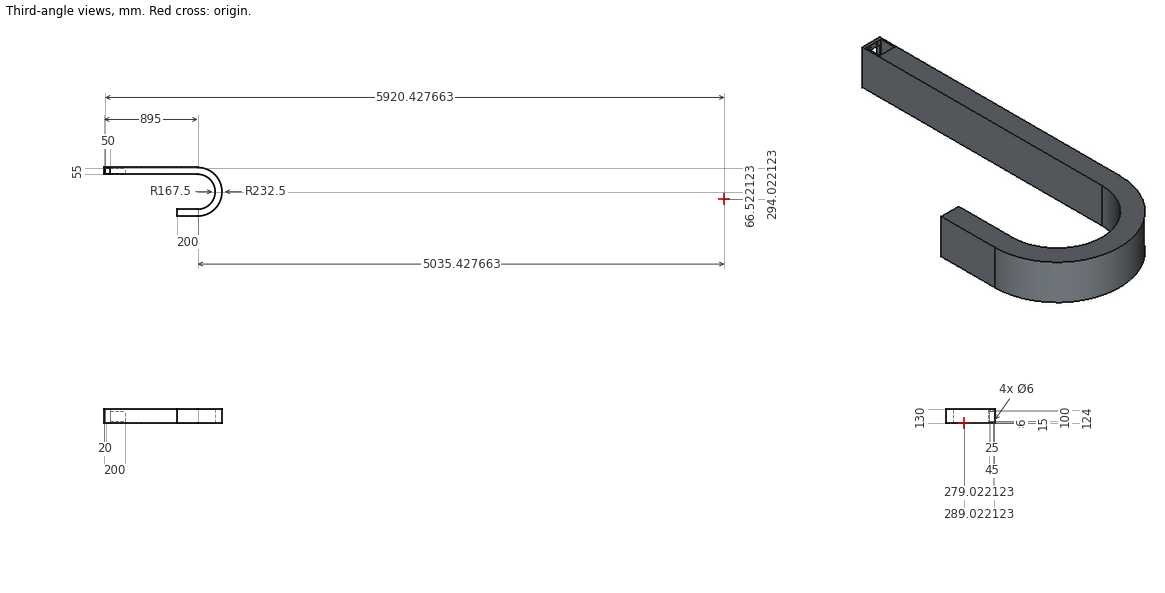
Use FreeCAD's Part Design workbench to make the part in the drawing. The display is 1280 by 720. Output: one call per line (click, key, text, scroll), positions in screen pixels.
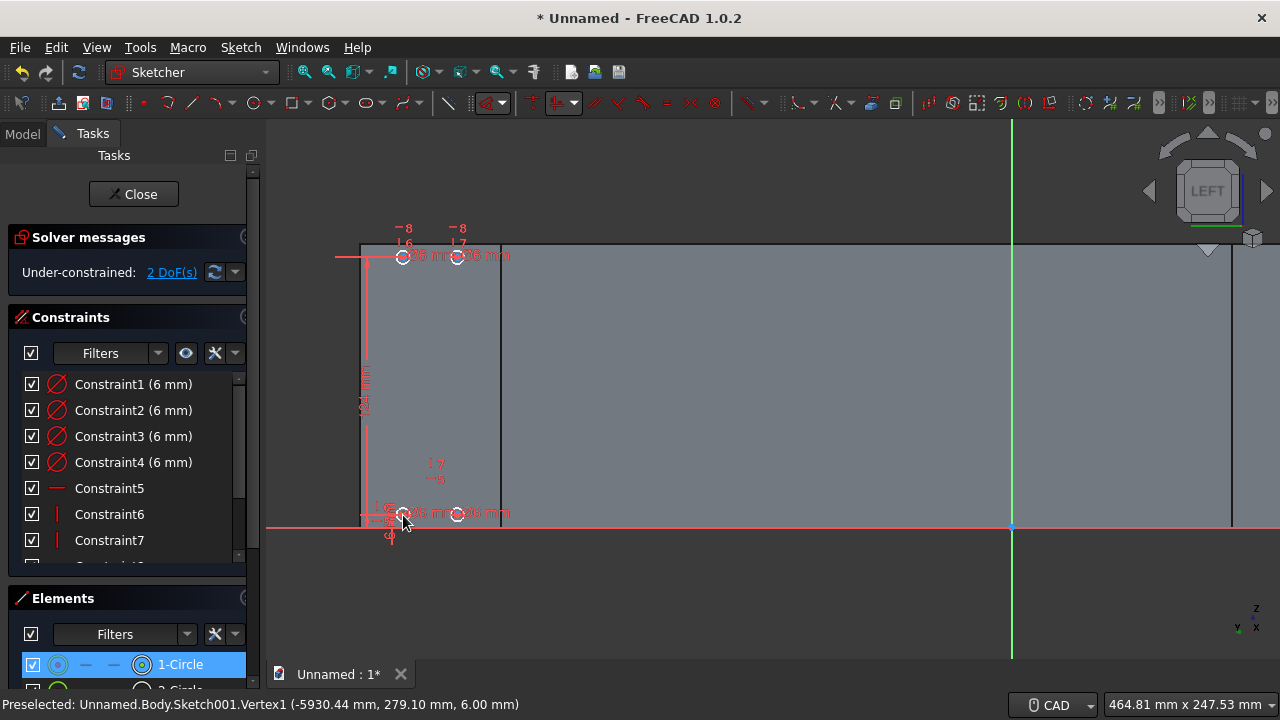
click(457, 515)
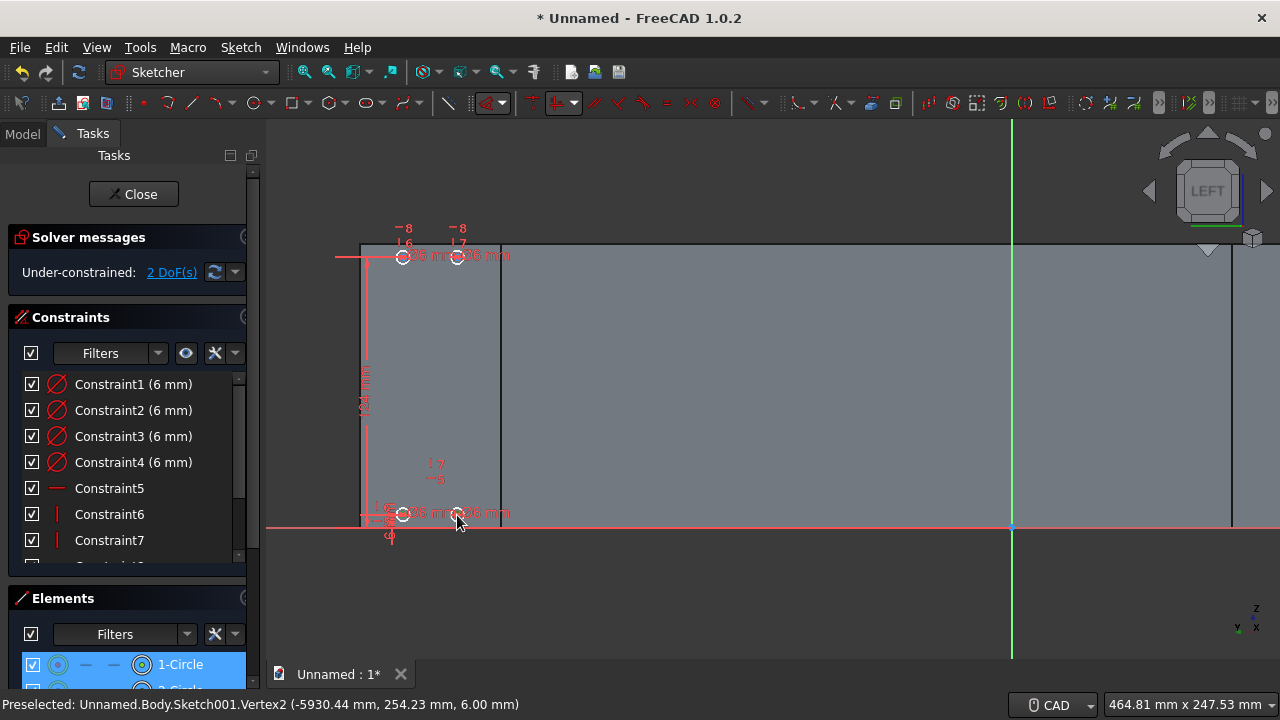
key(l)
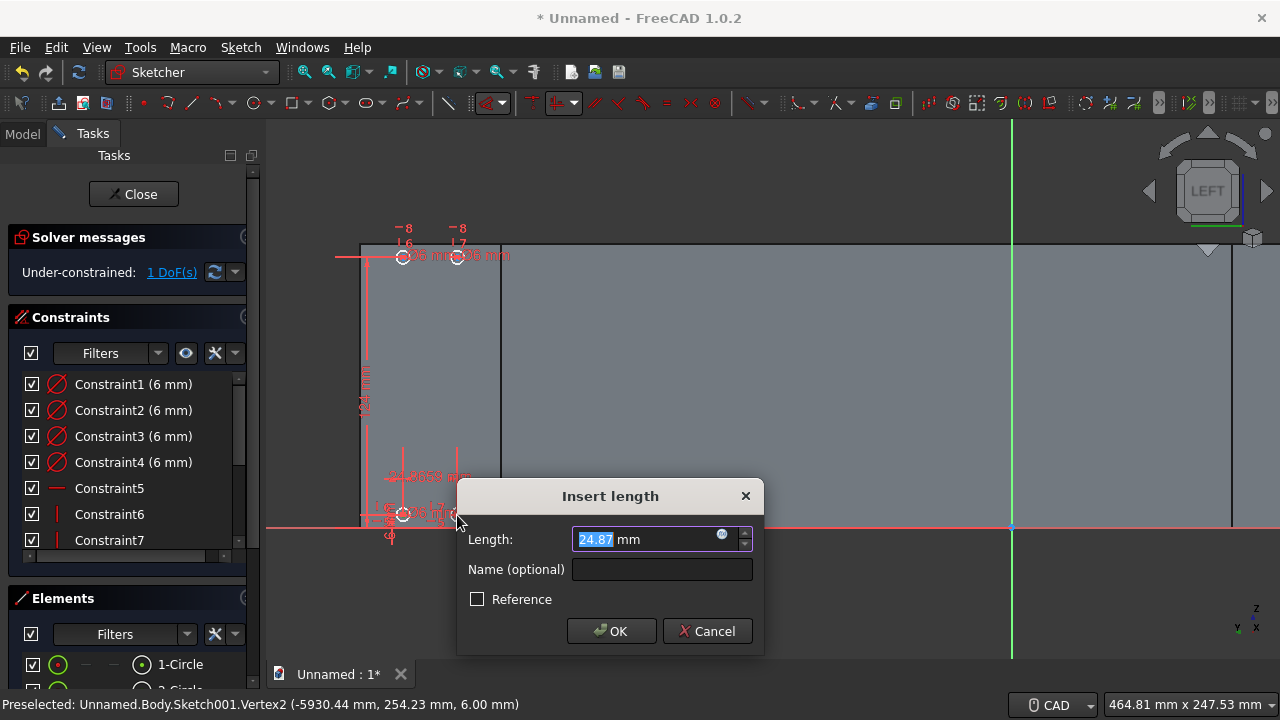
text(25)
key(Return)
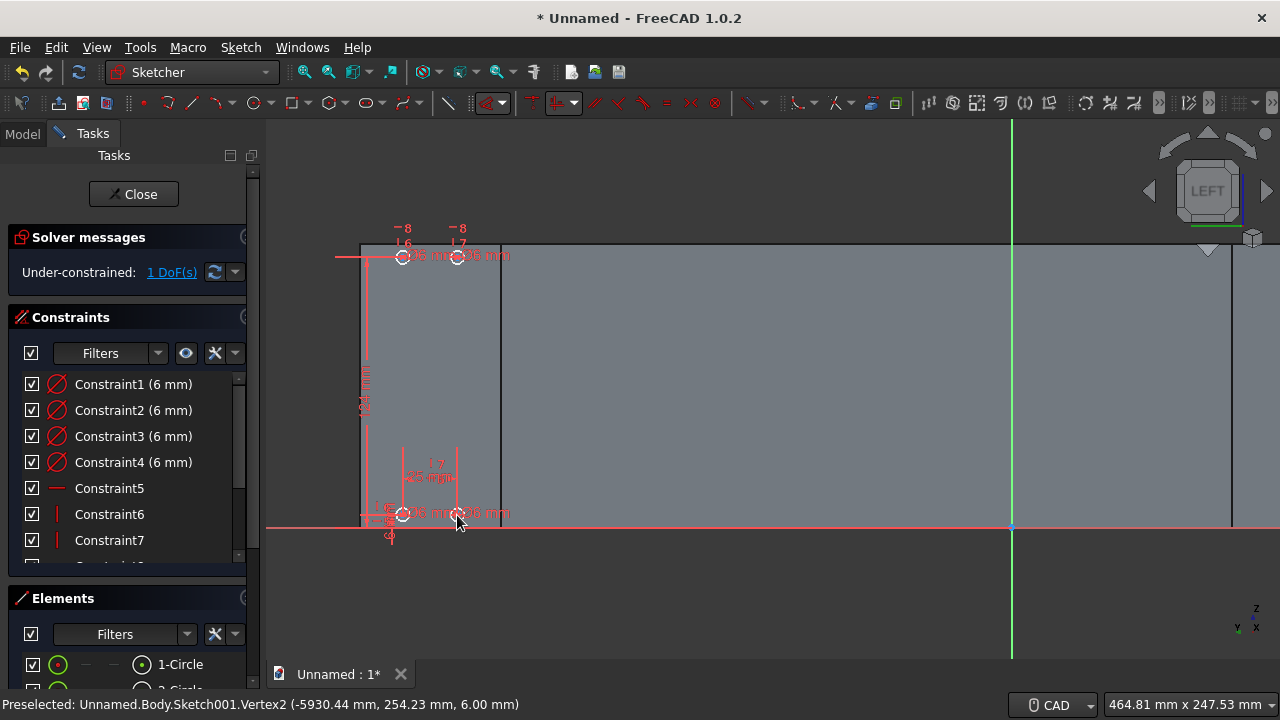
click(403, 515)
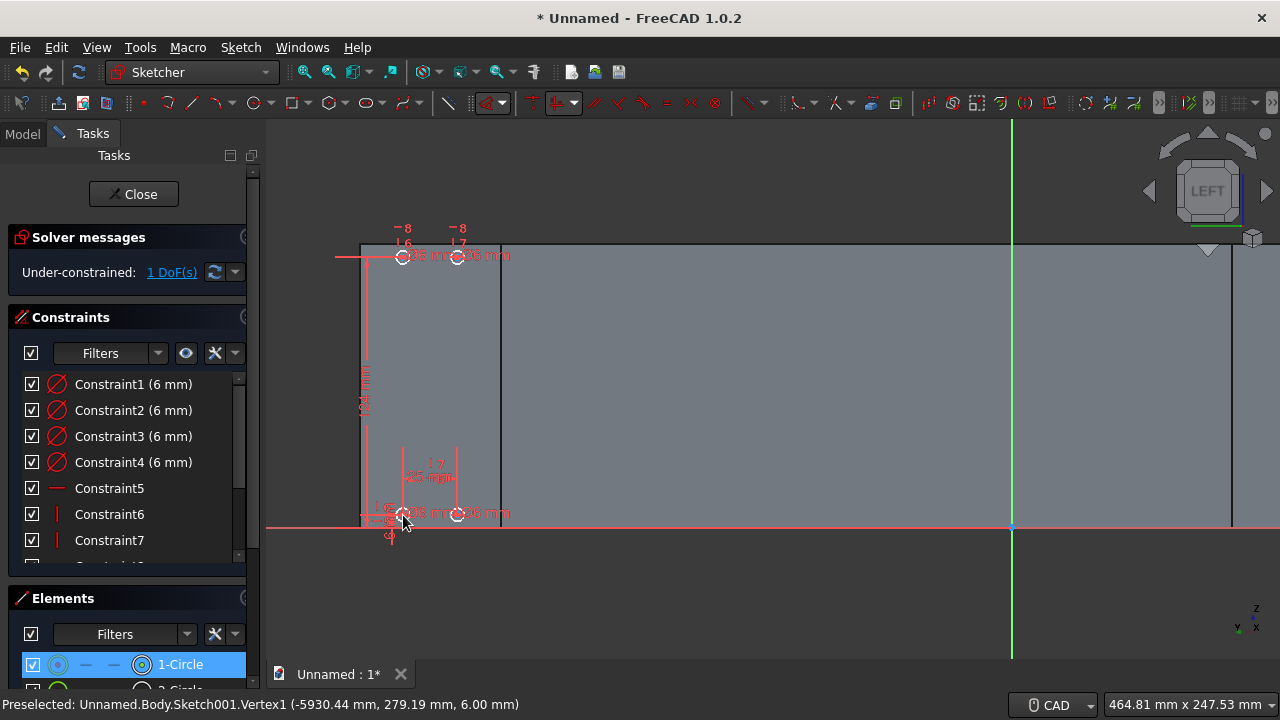
key(l)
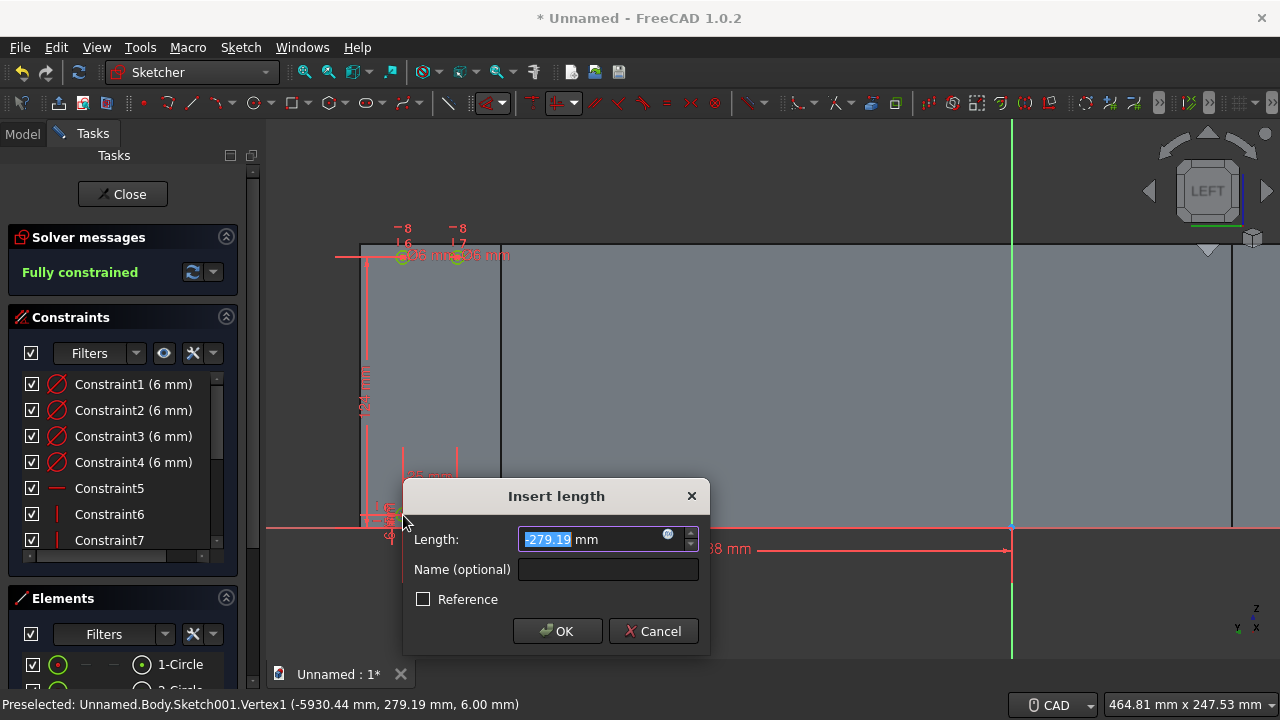
text(-279.022123)
key(Return)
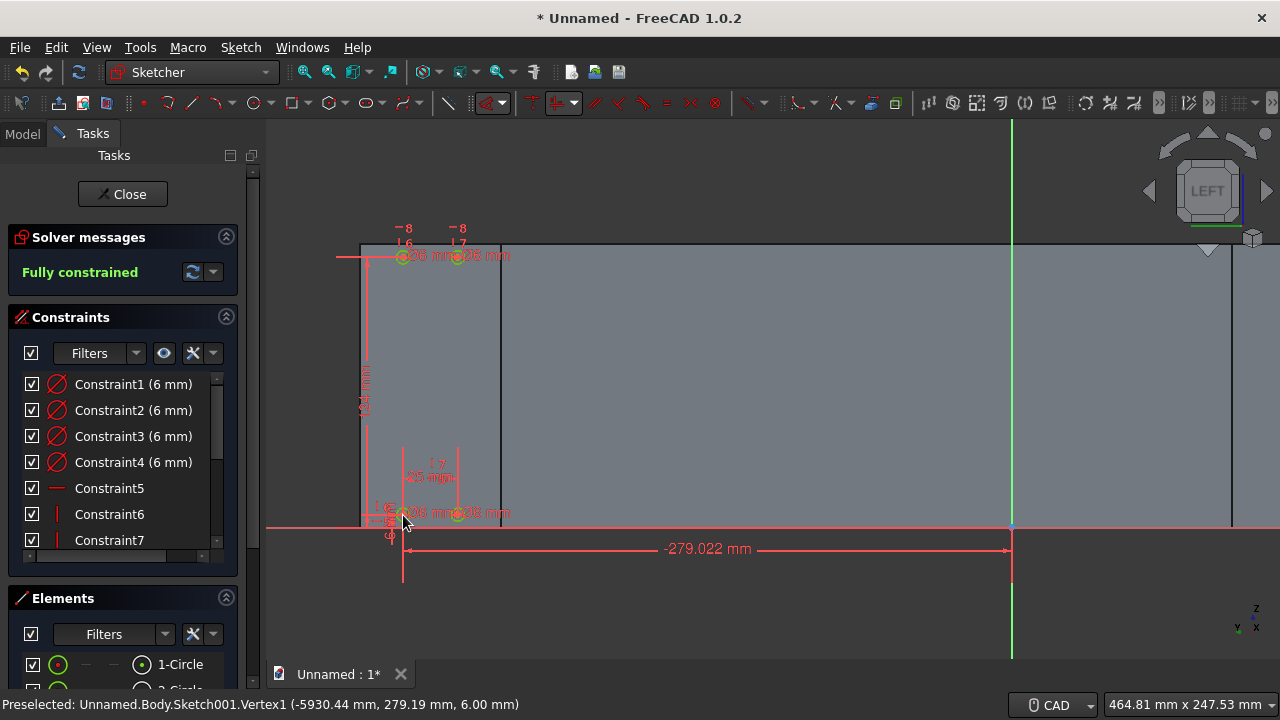
click(123, 194)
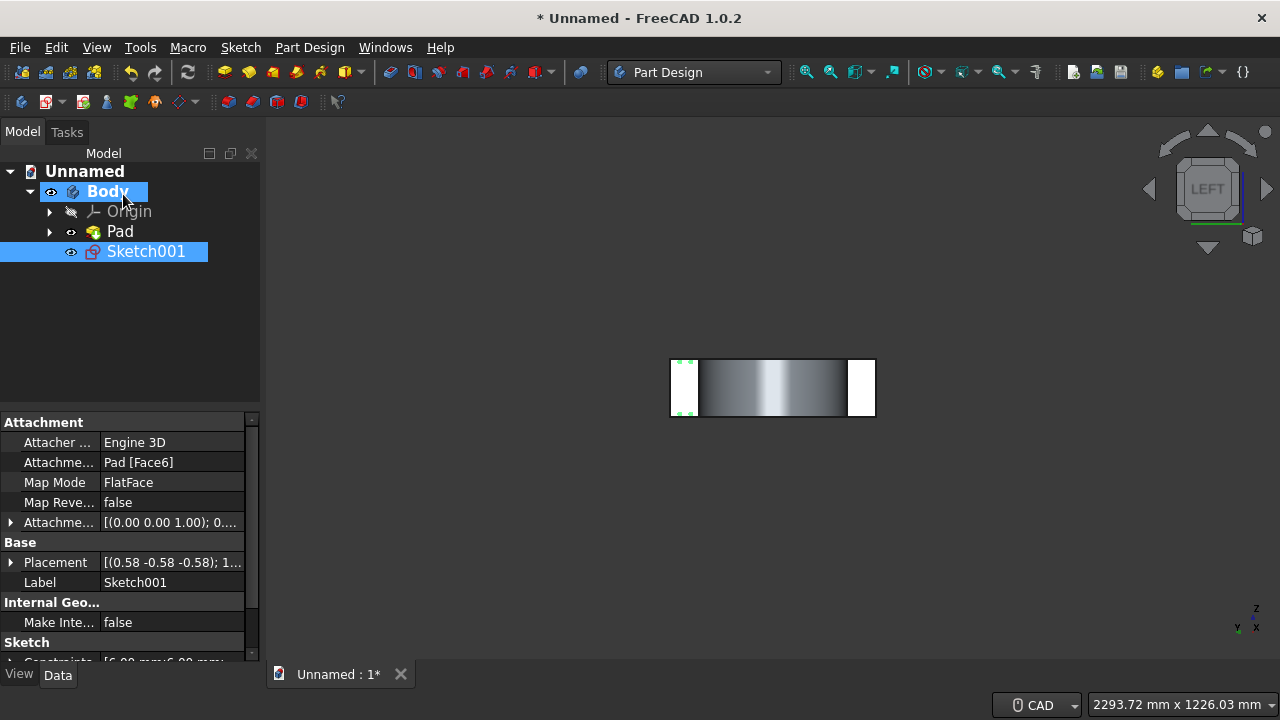
click(392, 72)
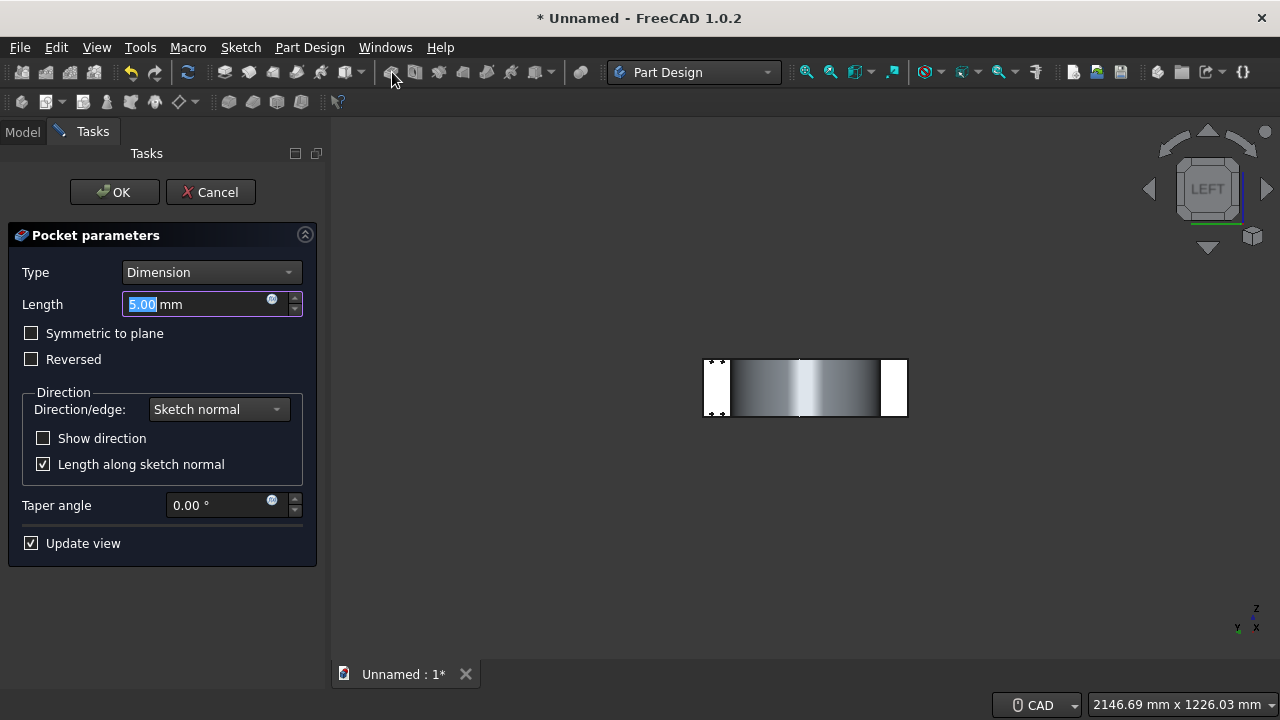
text(20)
key(Tab)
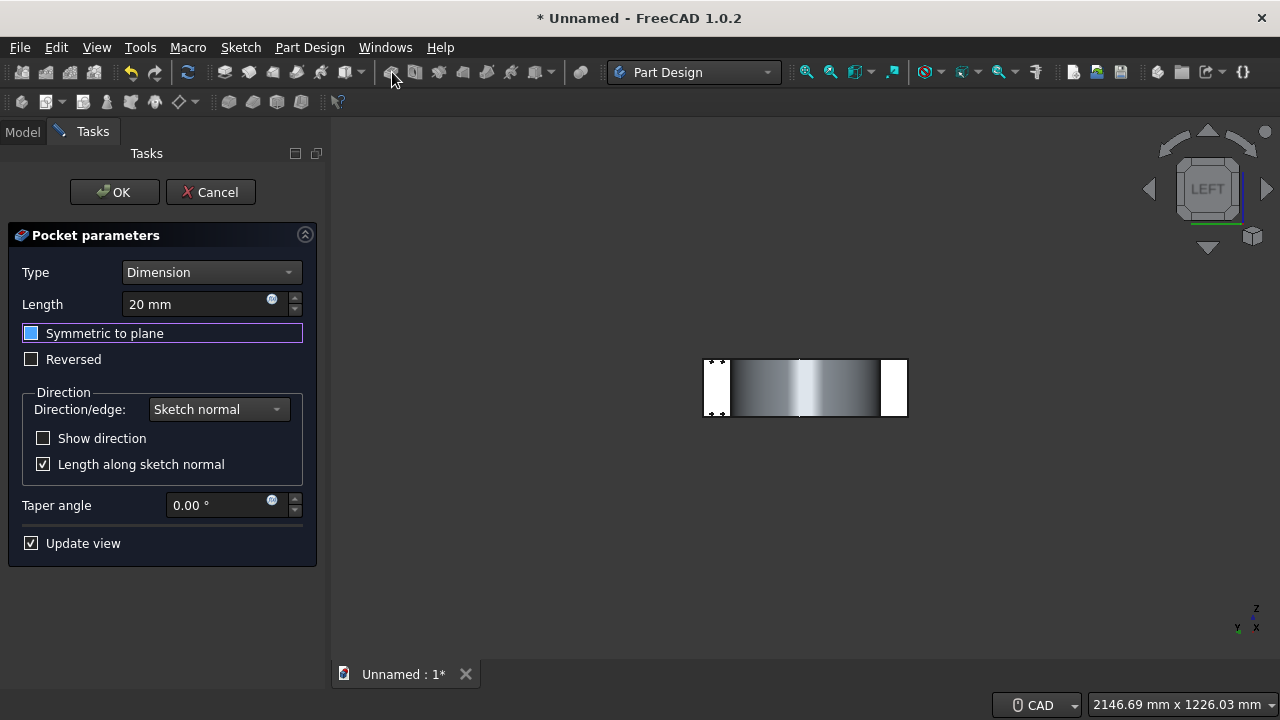
click(115, 192)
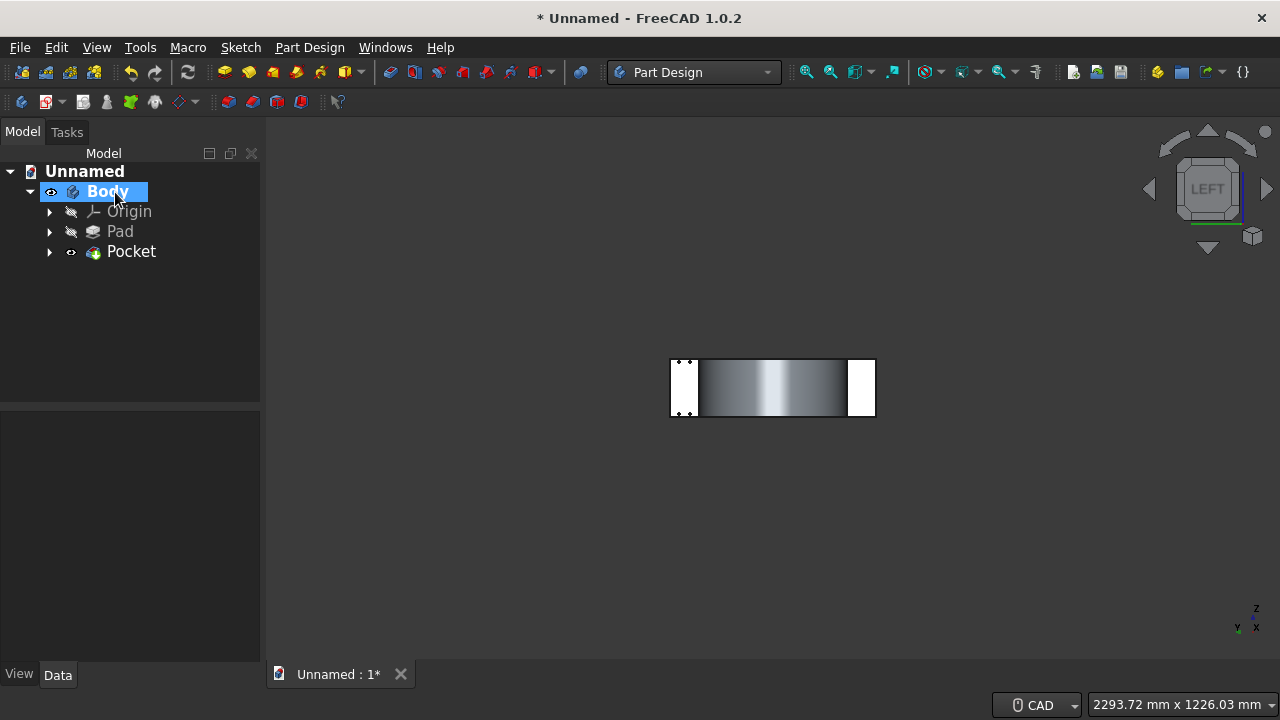
click(808, 72)